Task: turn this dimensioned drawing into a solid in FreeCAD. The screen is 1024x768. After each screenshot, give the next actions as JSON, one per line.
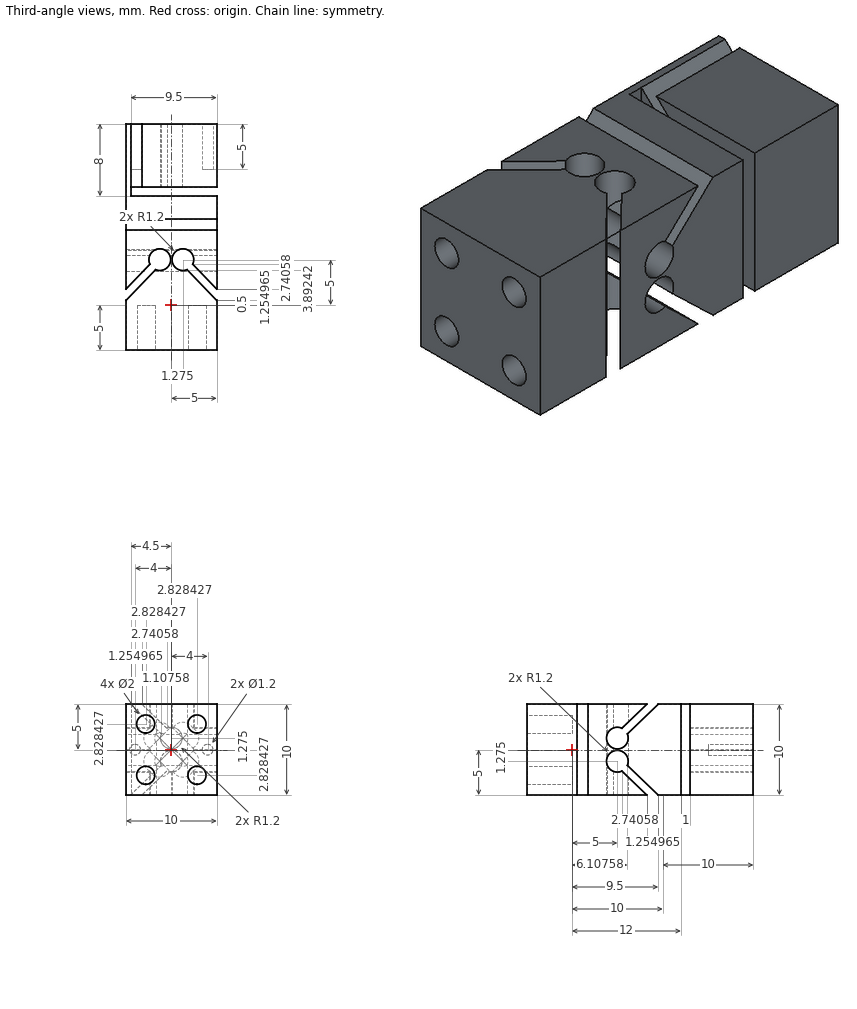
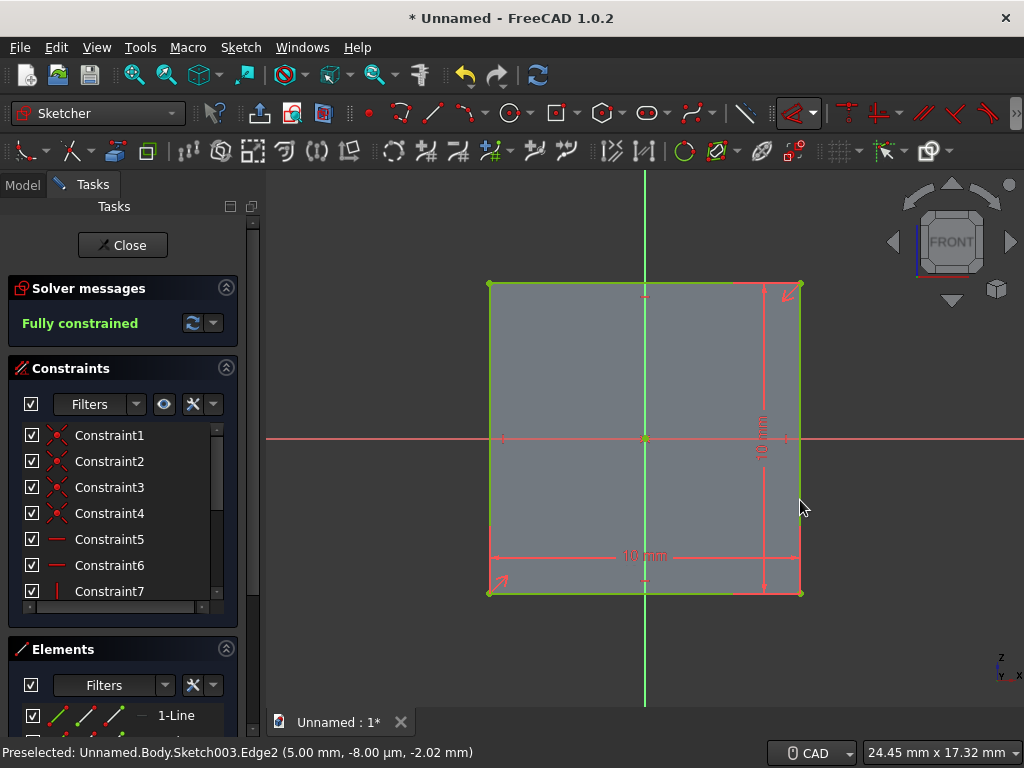
{"action": "left_click", "coordinate": [123, 245]}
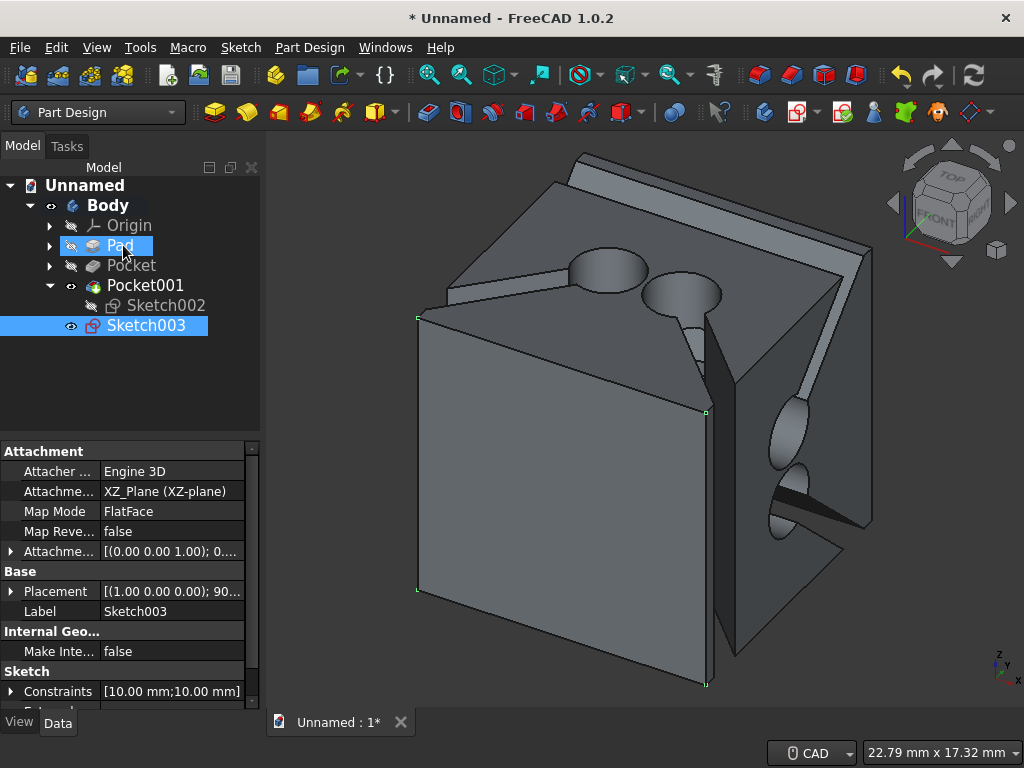
{"action": "left_click", "coordinate": [216, 112]}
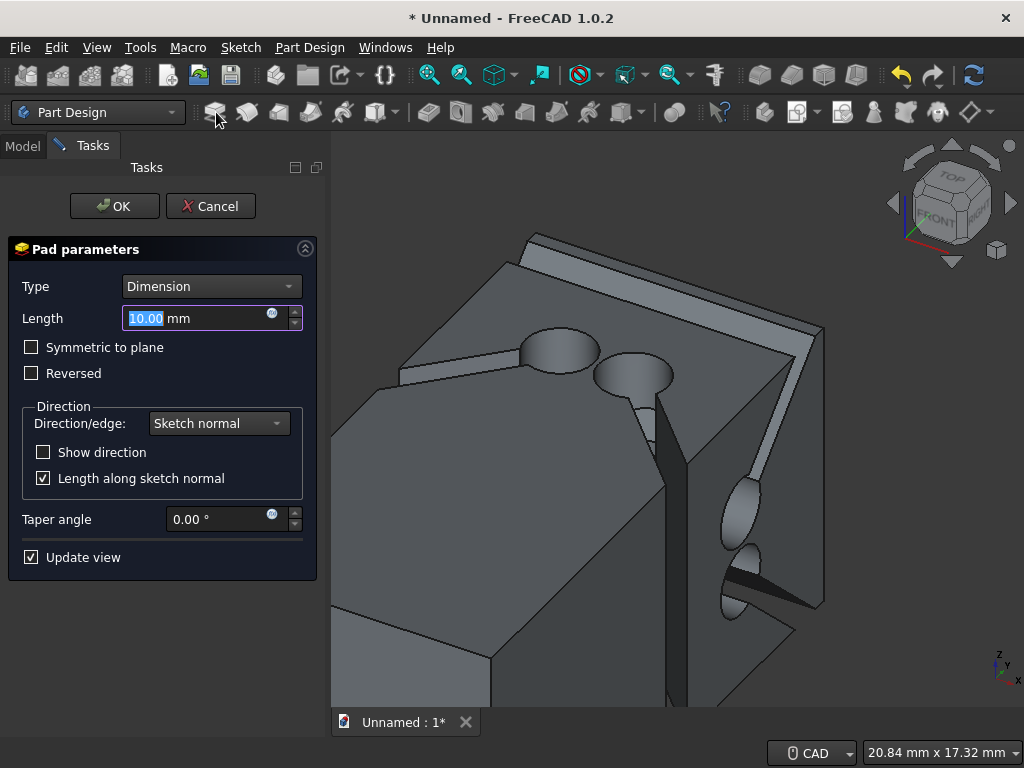
{"action": "type", "text": "5"}
{"action": "key", "text": "Tab"}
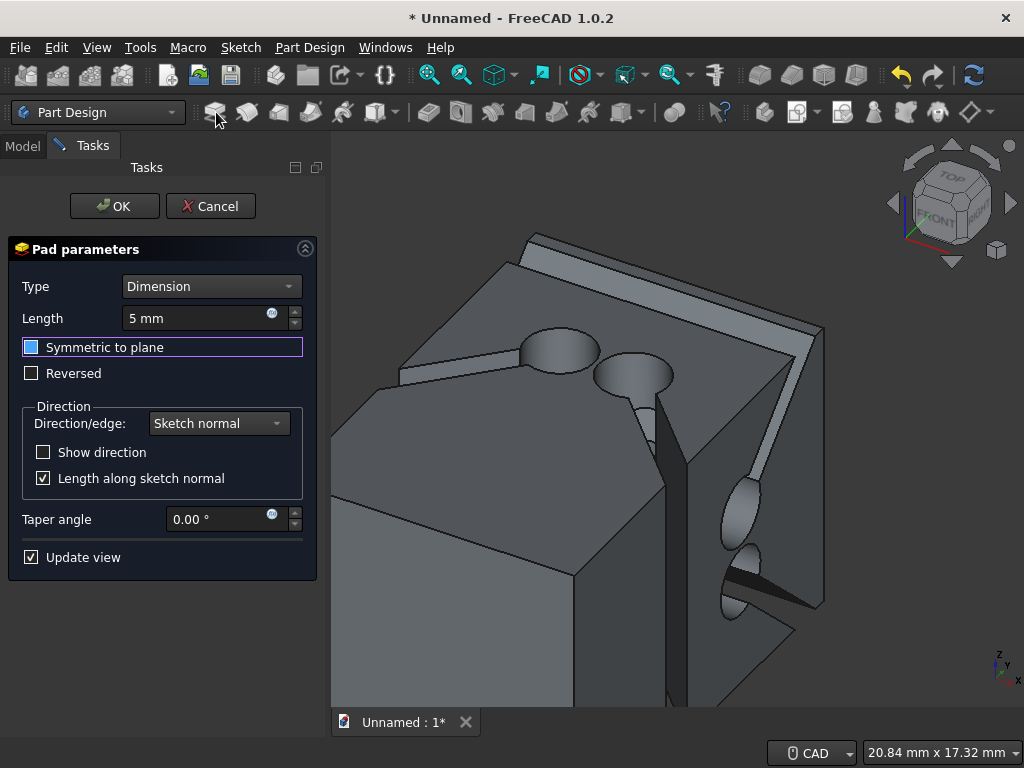
{"action": "left_click", "coordinate": [115, 206]}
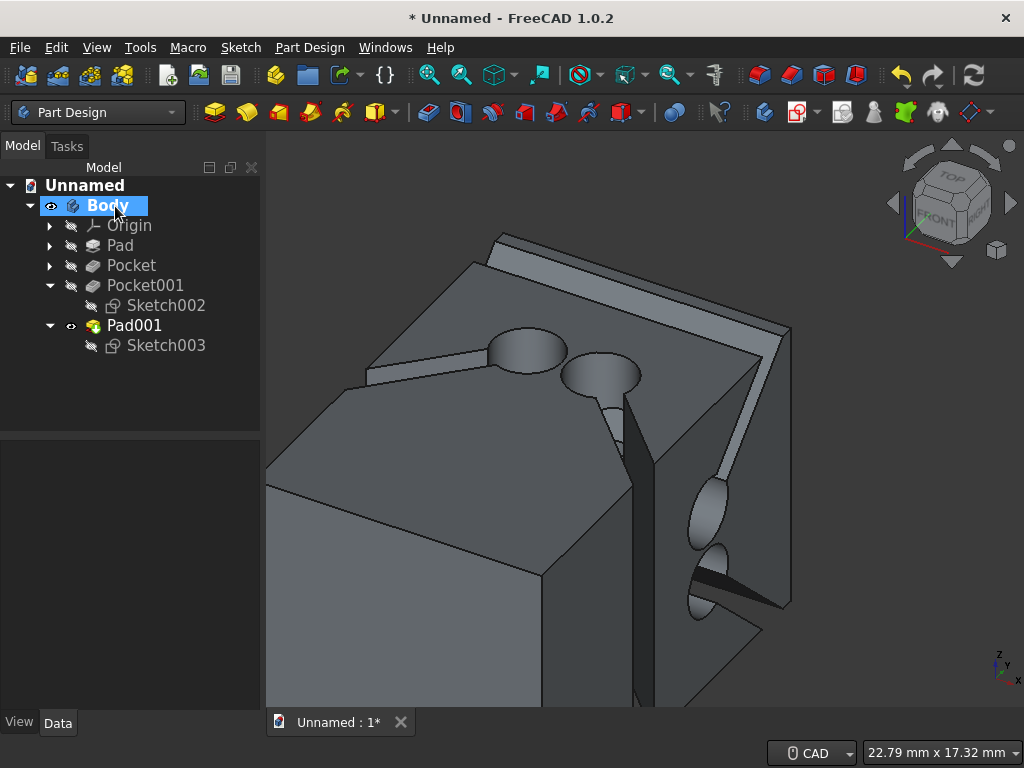
{"action": "key", "text": "v f"}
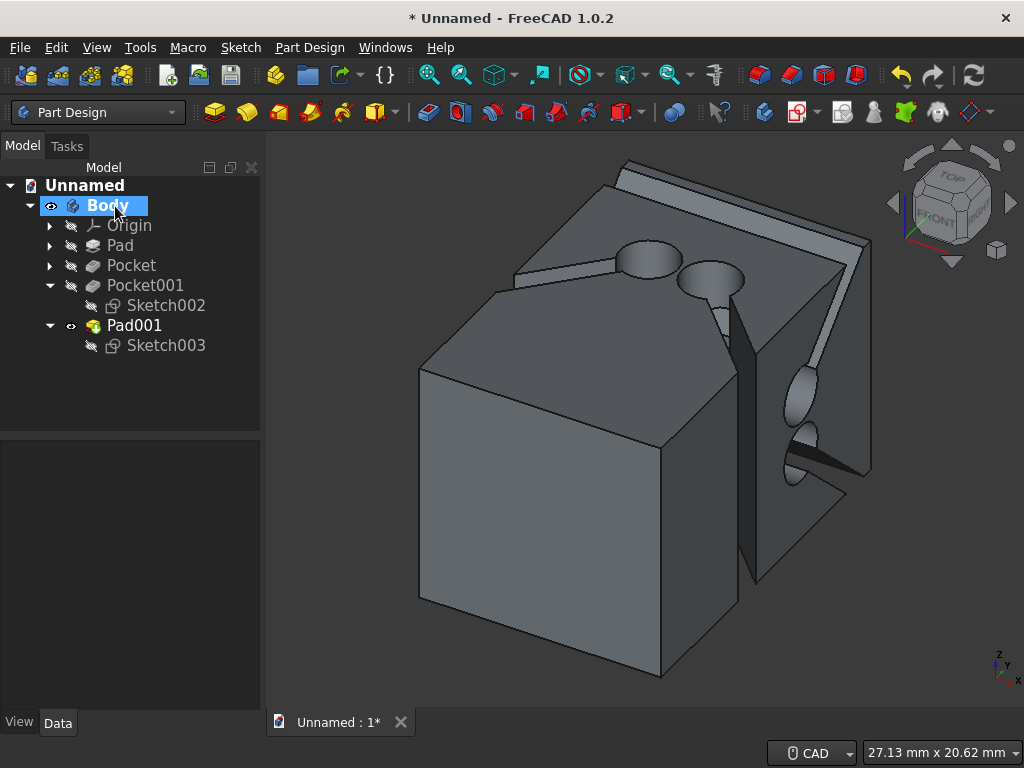
{"action": "key", "text": "4"}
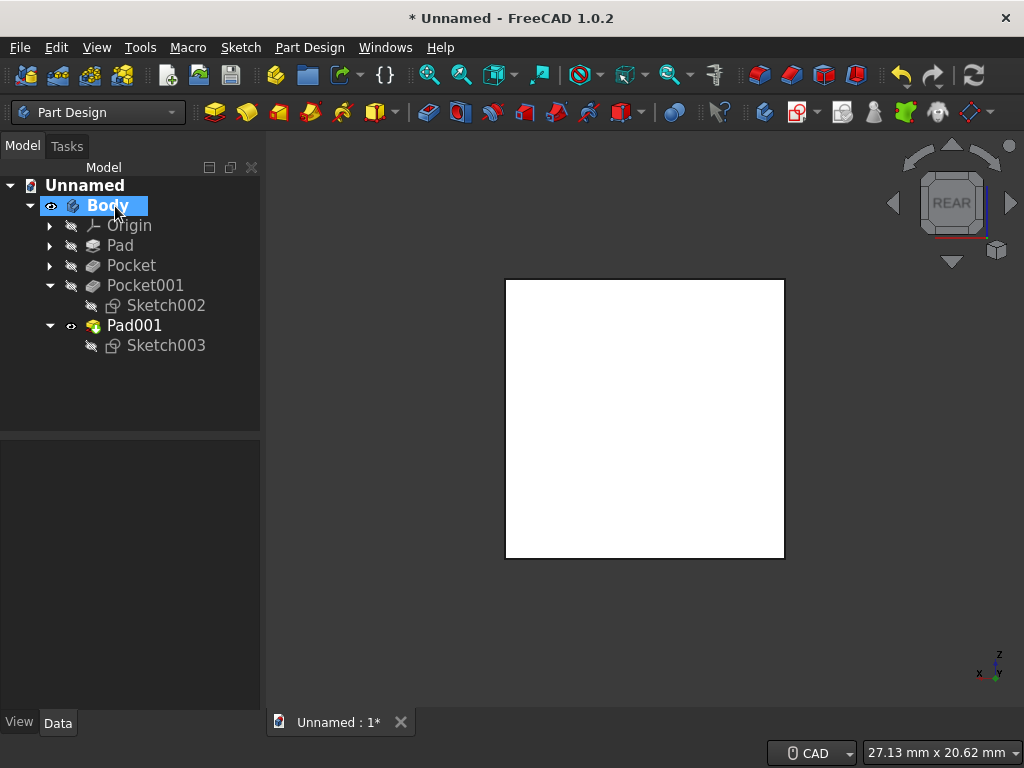
{"action": "left_click", "coordinate": [645, 418]}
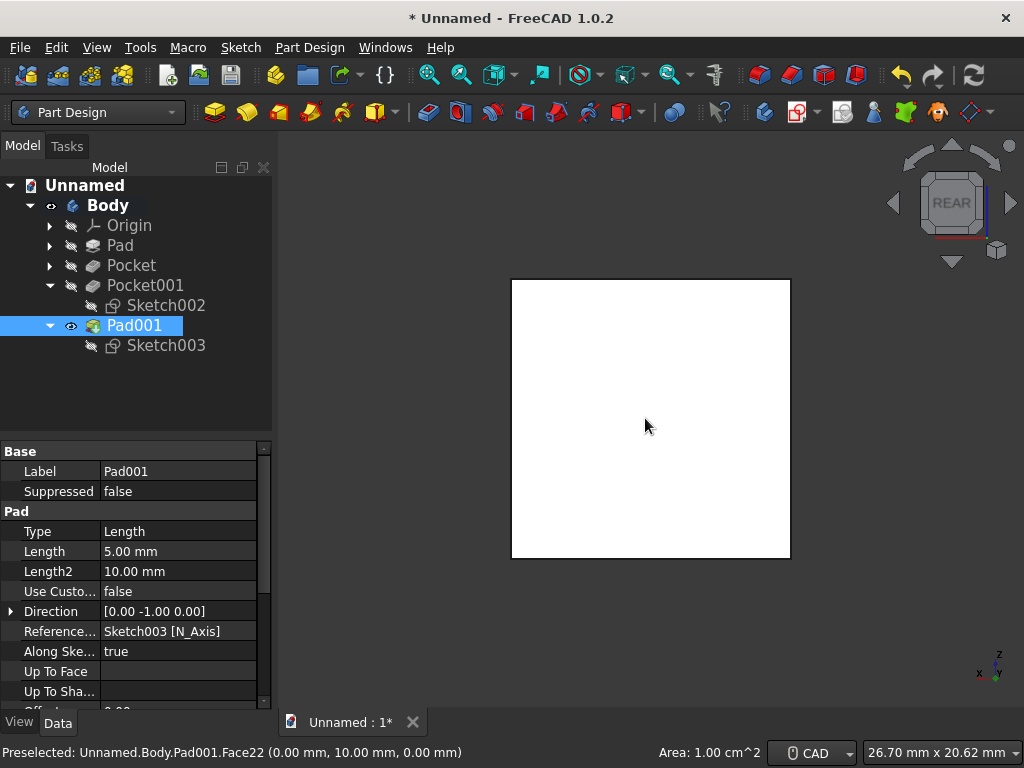
{"action": "left_click", "coordinate": [798, 112]}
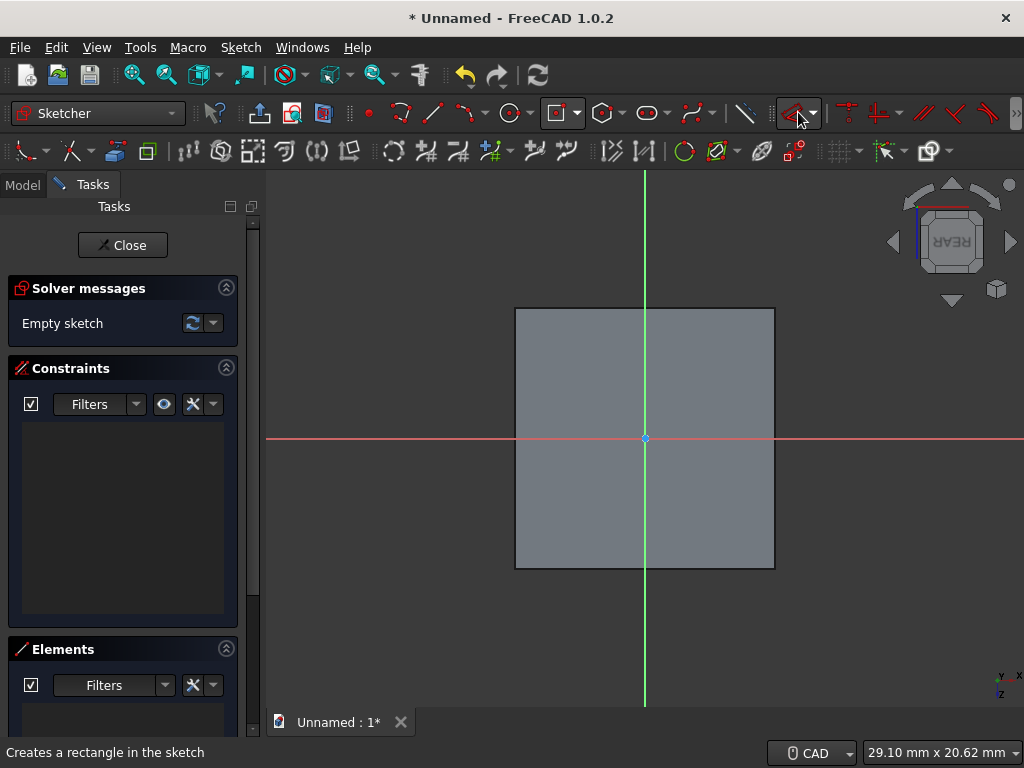
{"action": "left_click", "coordinate": [556, 114]}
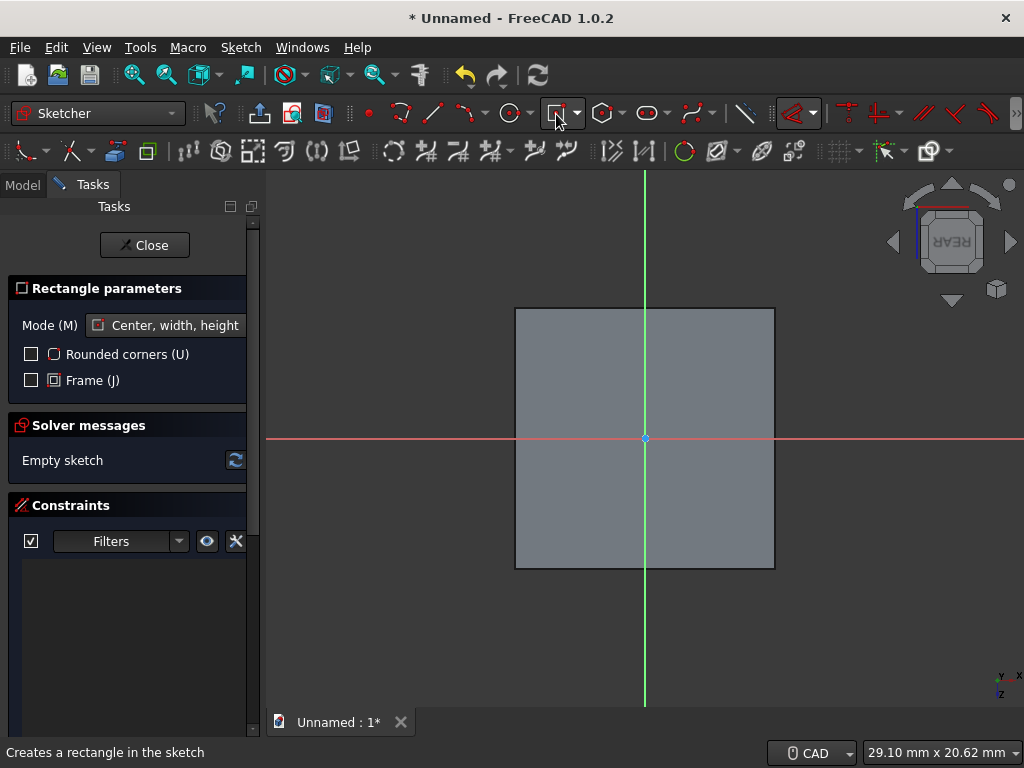
{"action": "left_click", "coordinate": [645, 439]}
{"action": "left_click", "coordinate": [775, 308]}
{"action": "key", "text": "Escape"}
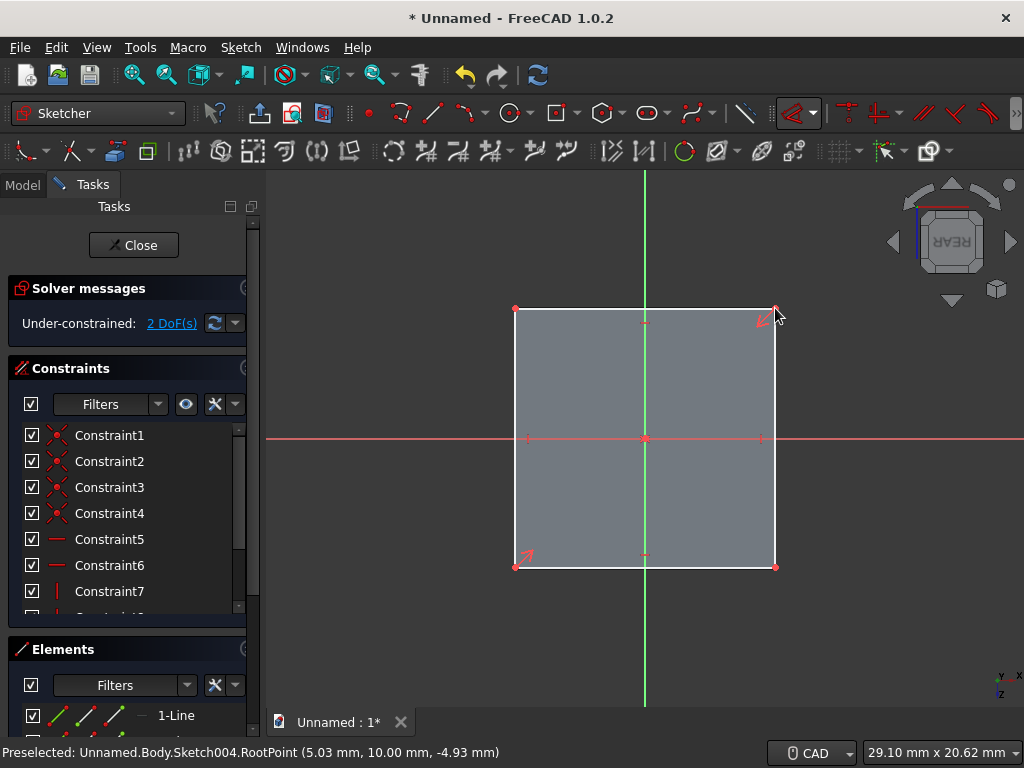
{"action": "left_click", "coordinate": [593, 568]}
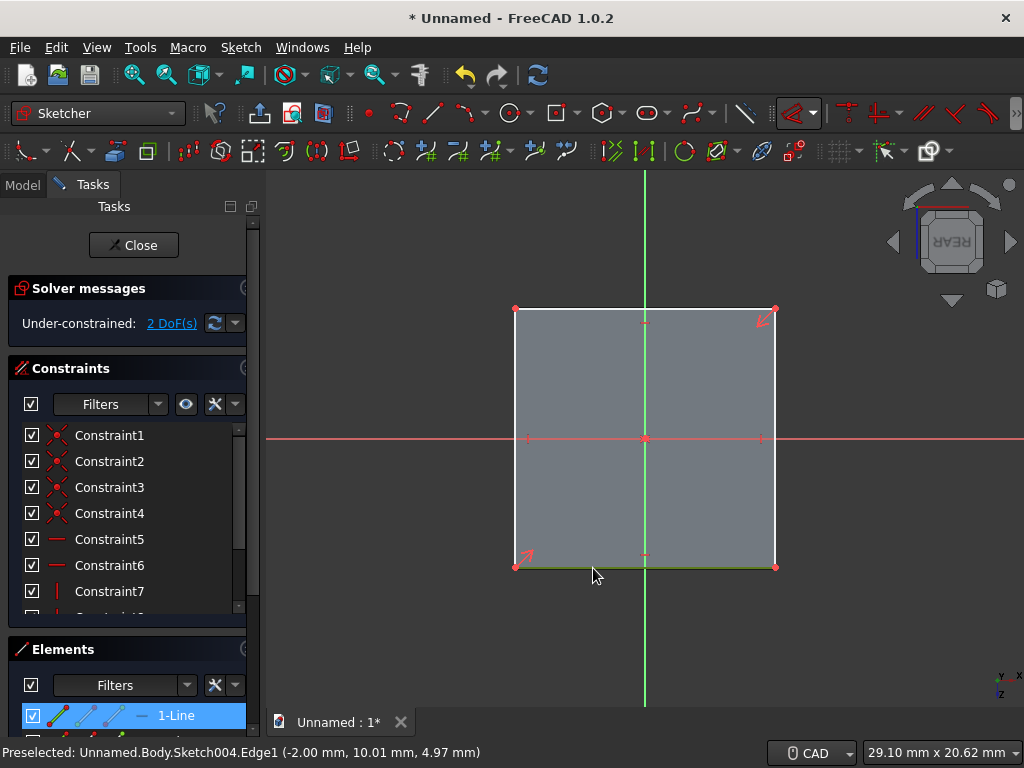
{"action": "key", "text": "l"}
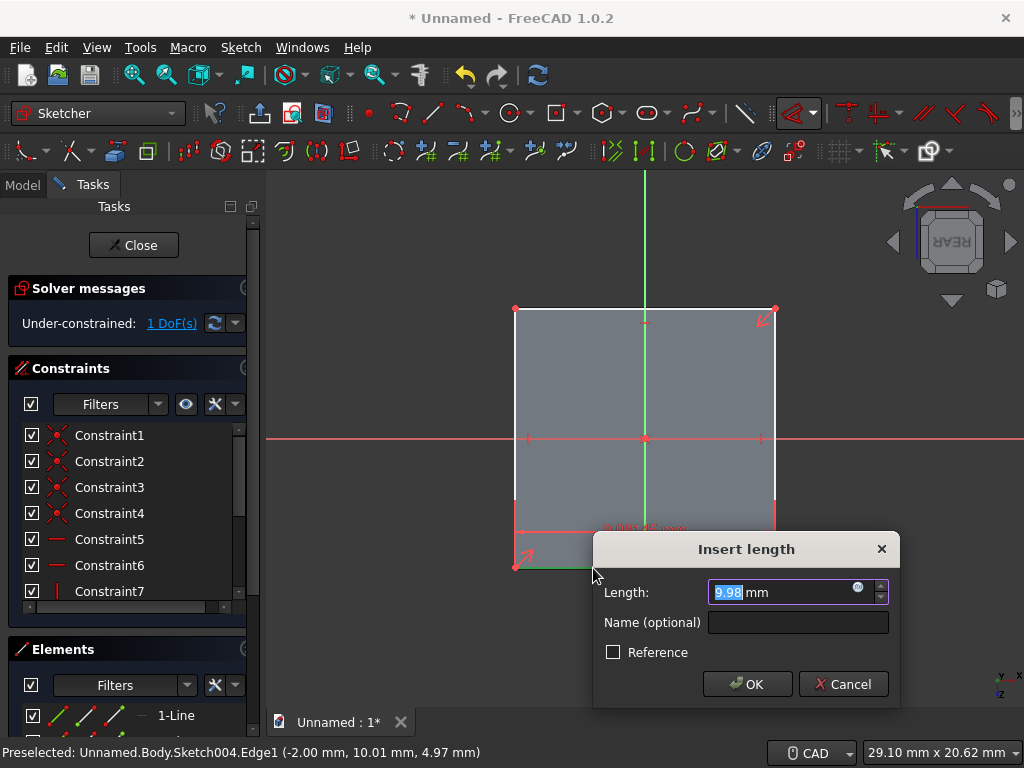
{"action": "type", "text": "10"}
{"action": "key", "text": "Return"}